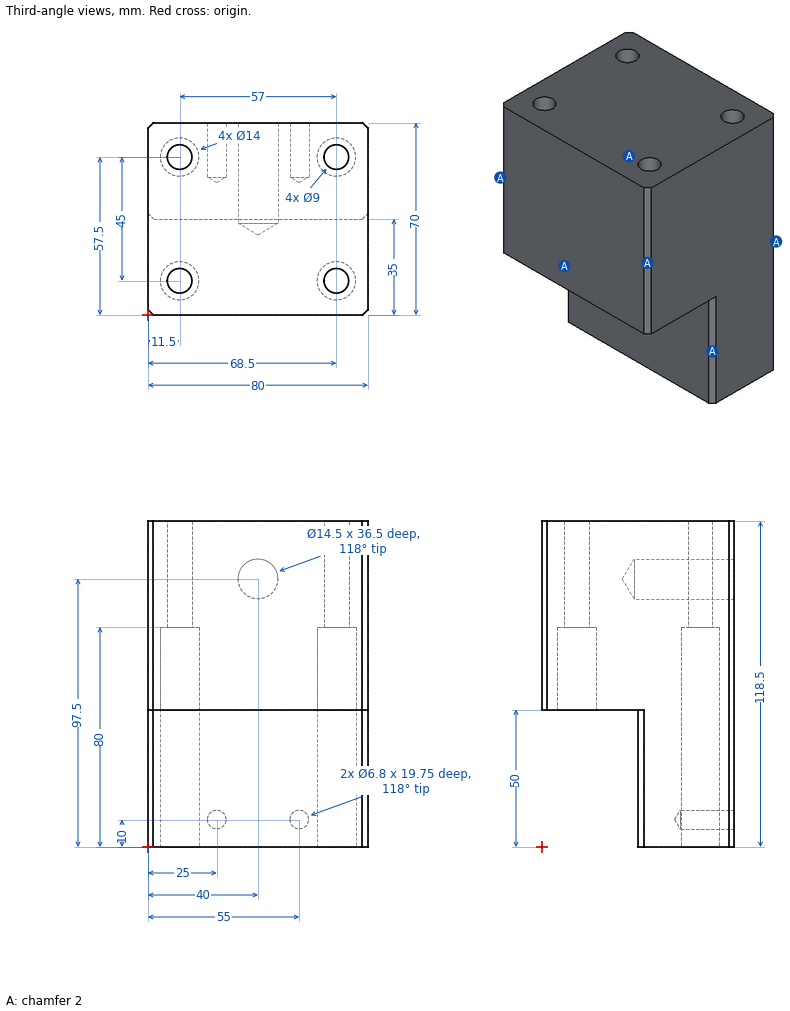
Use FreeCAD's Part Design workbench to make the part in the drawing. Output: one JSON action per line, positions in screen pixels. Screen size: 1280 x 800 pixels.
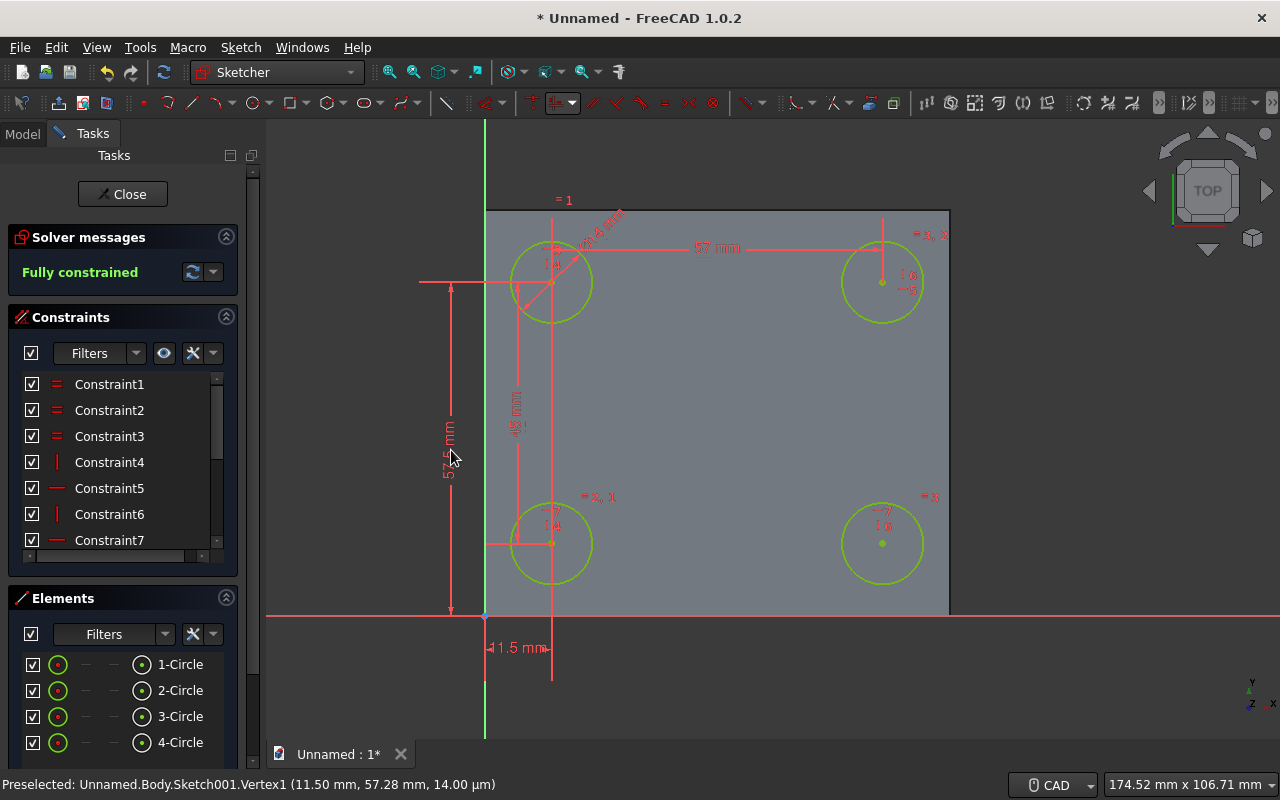
{"action": "left_click", "coordinate": [123, 194]}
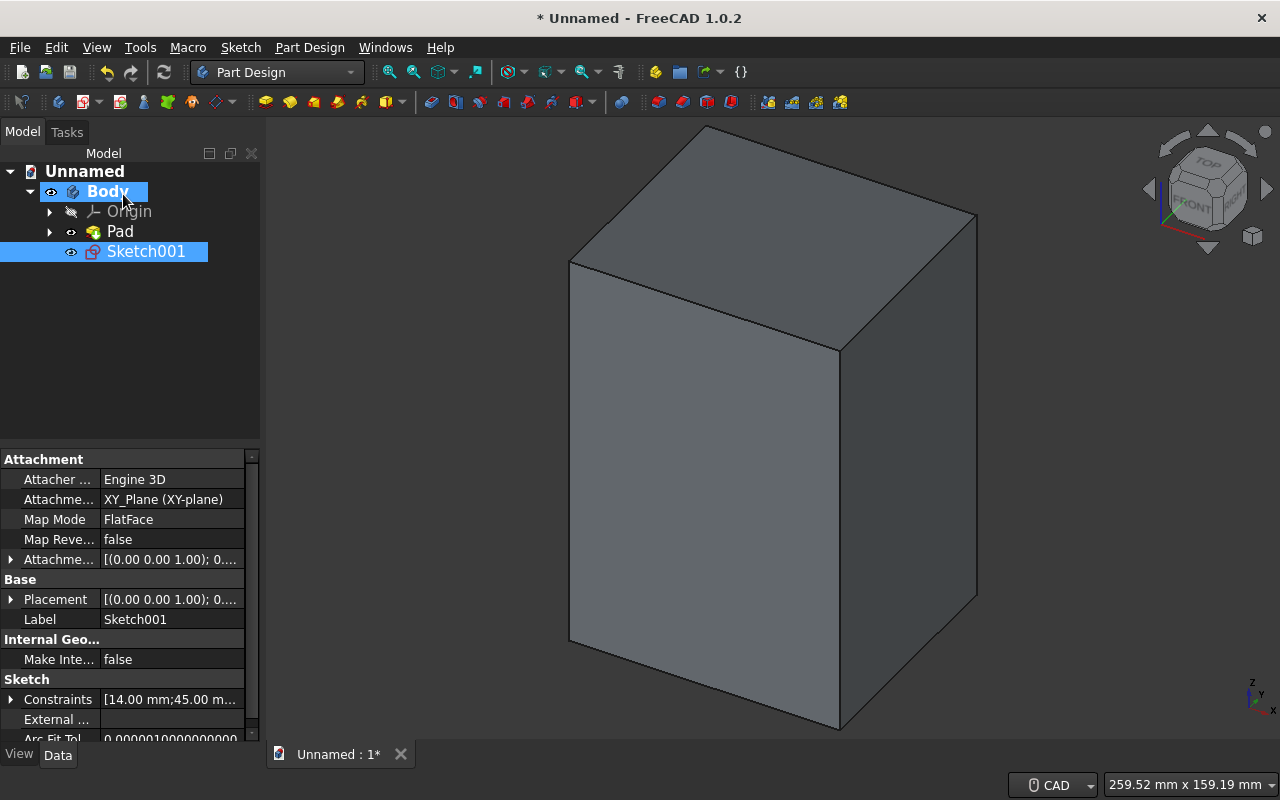
{"action": "left_click", "coordinate": [432, 102]}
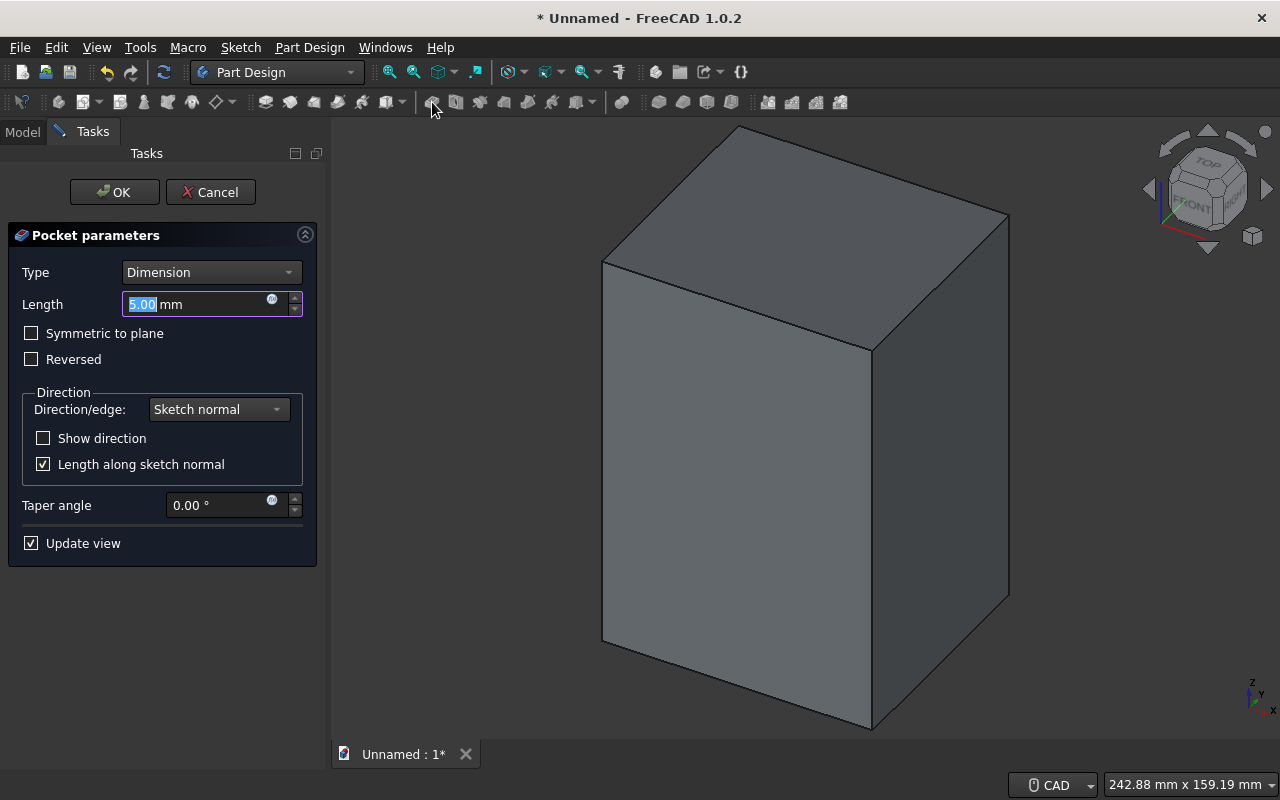
{"action": "type", "text": "80"}
{"action": "key", "text": "Tab"}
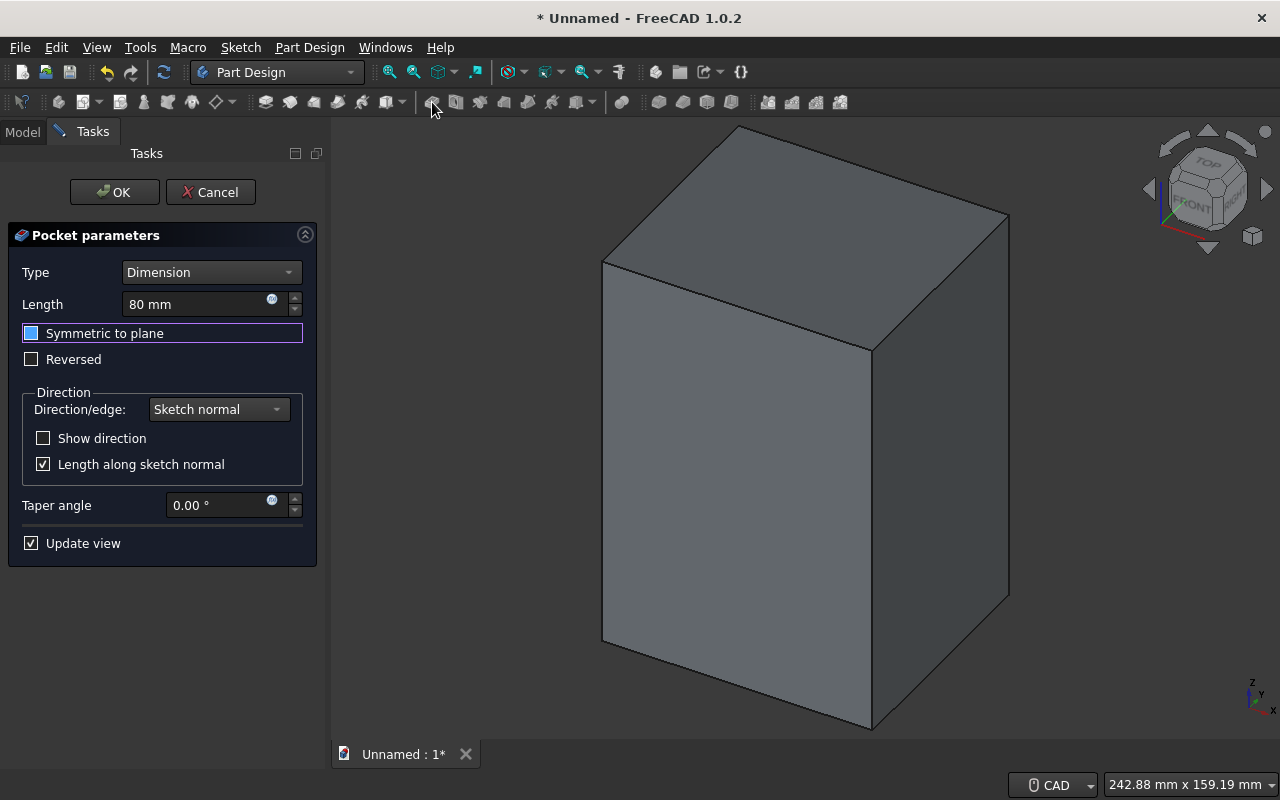
{"action": "left_click", "coordinate": [30, 359]}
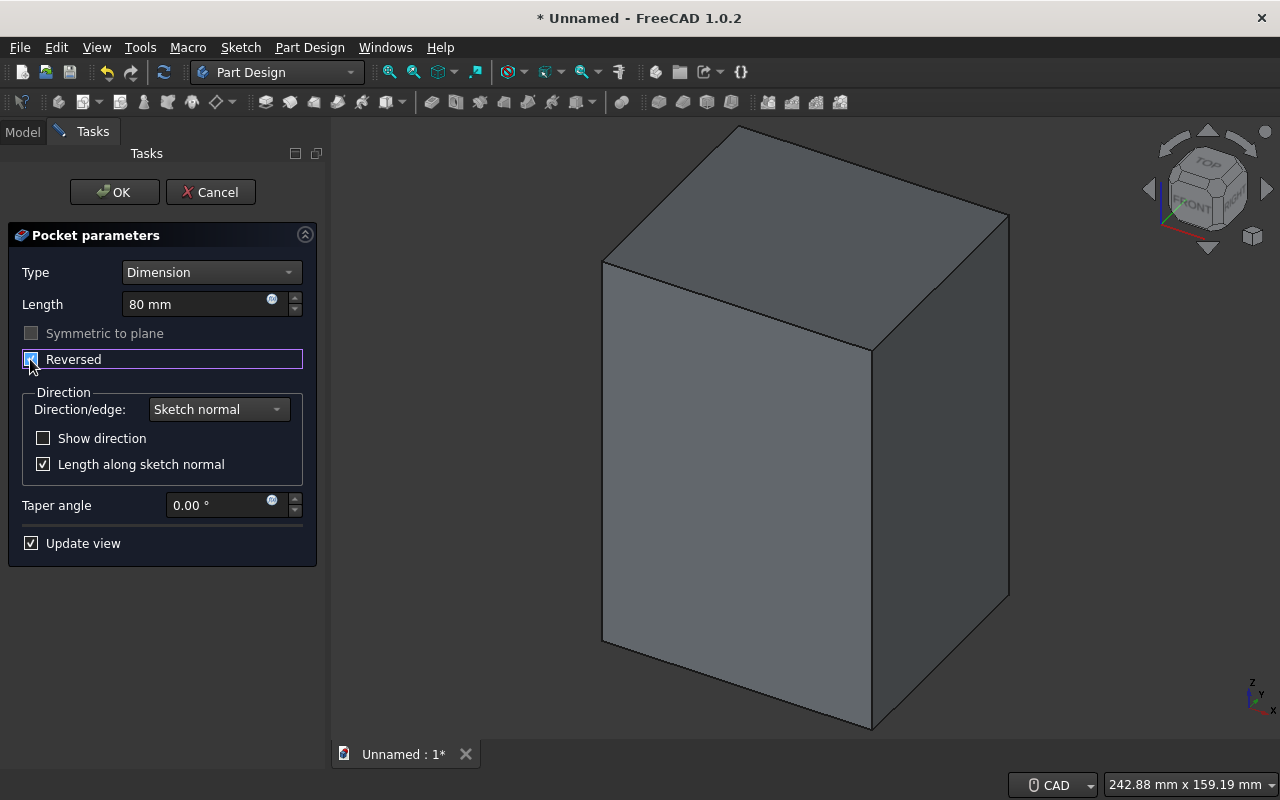
{"action": "left_click", "coordinate": [115, 192]}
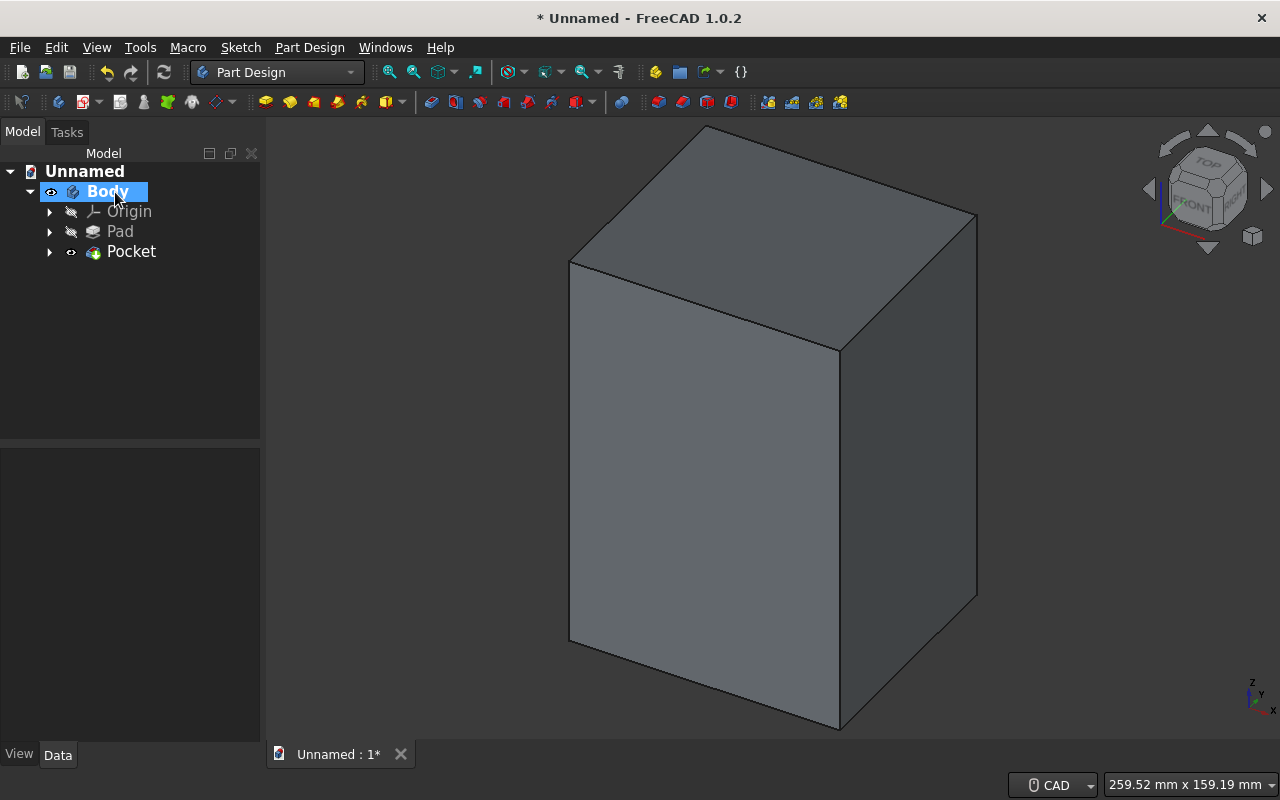
{"action": "left_click", "coordinate": [84, 102]}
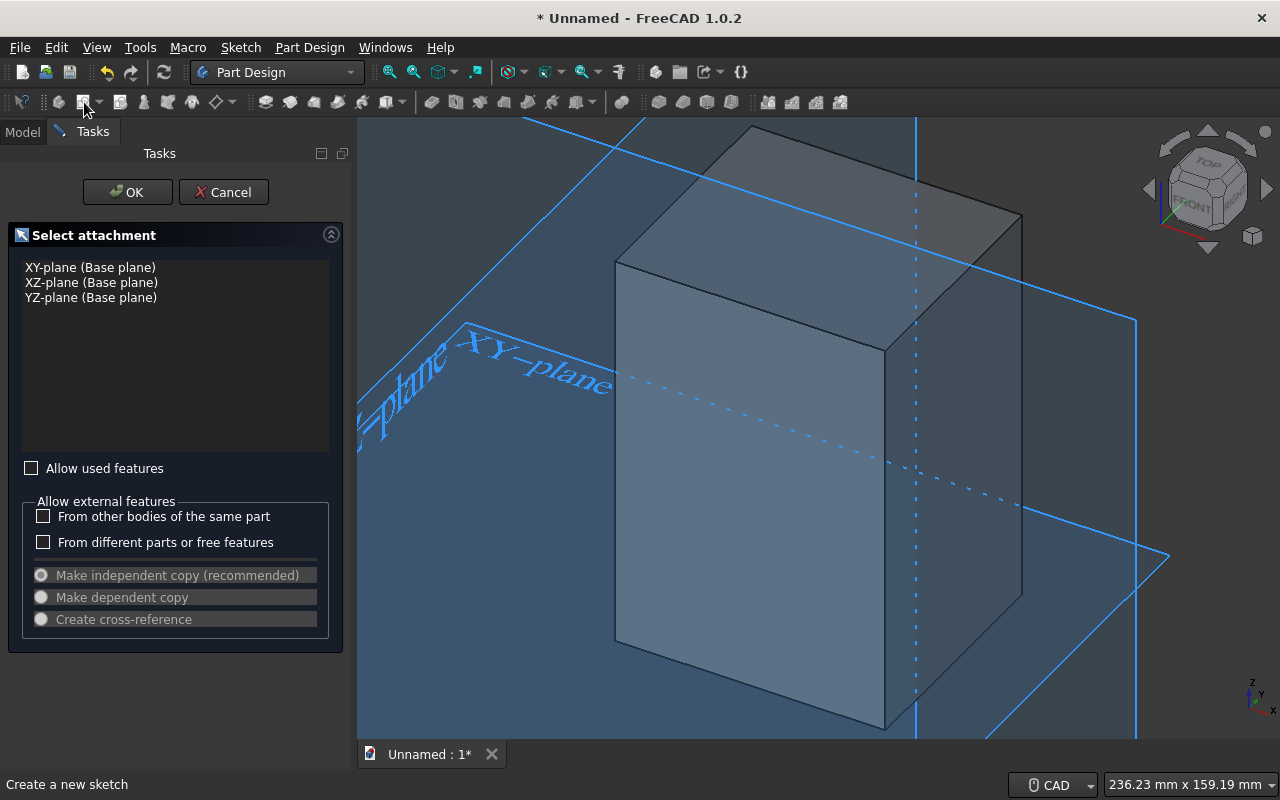
{"action": "left_click", "coordinate": [82, 268]}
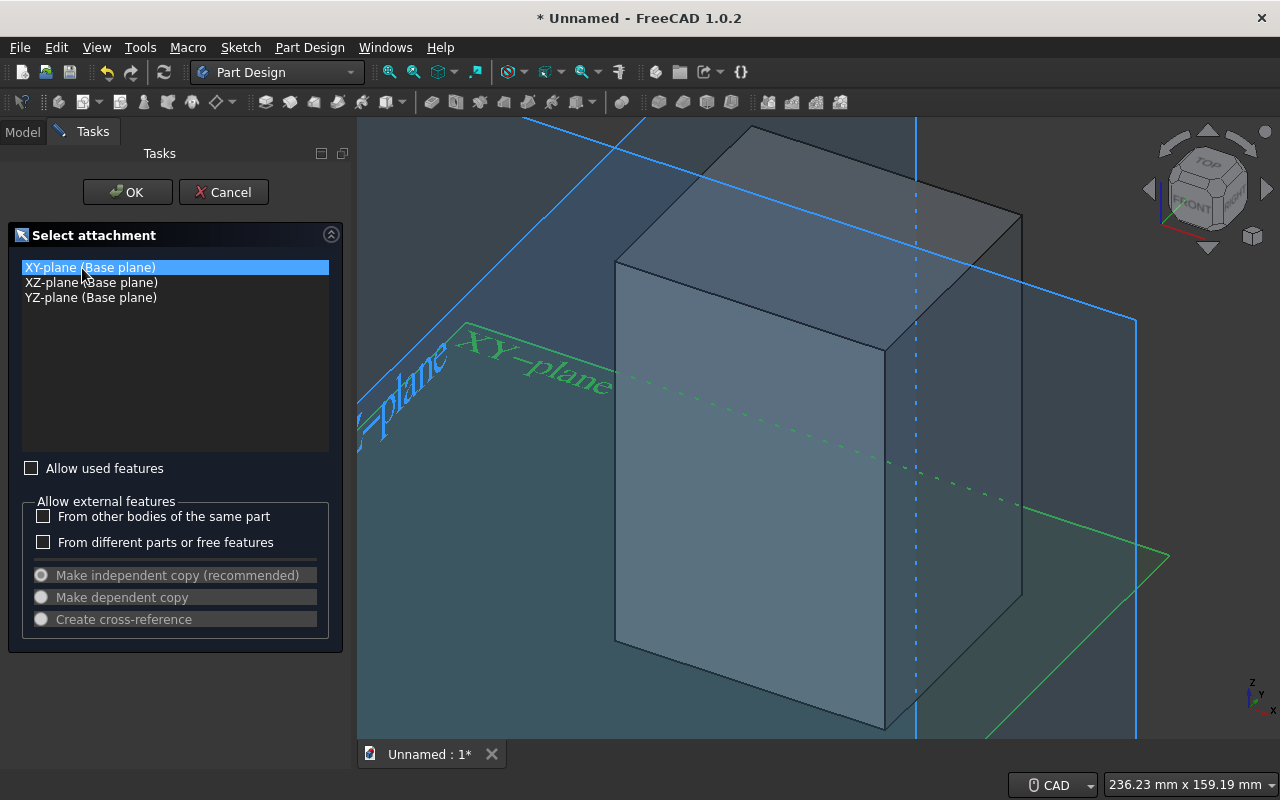
{"action": "left_click", "coordinate": [128, 192]}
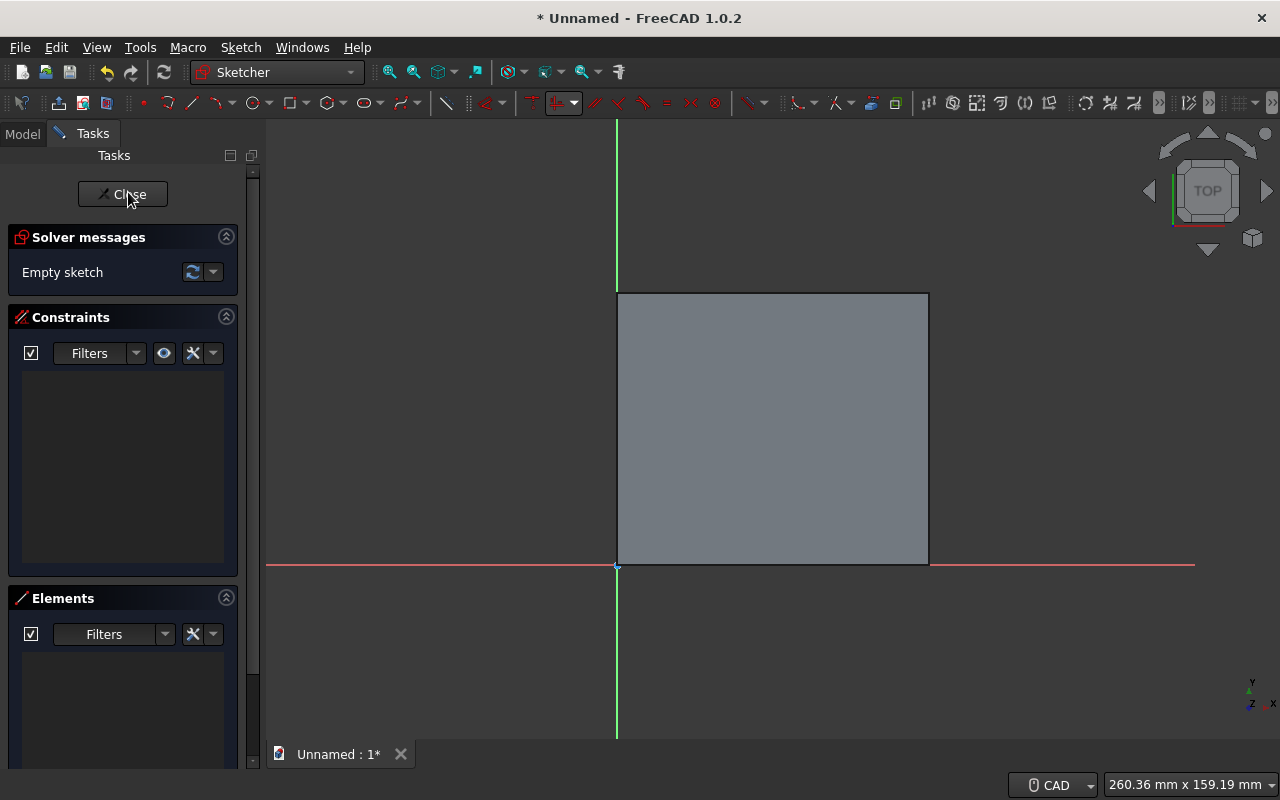
{"action": "key", "text": "q s"}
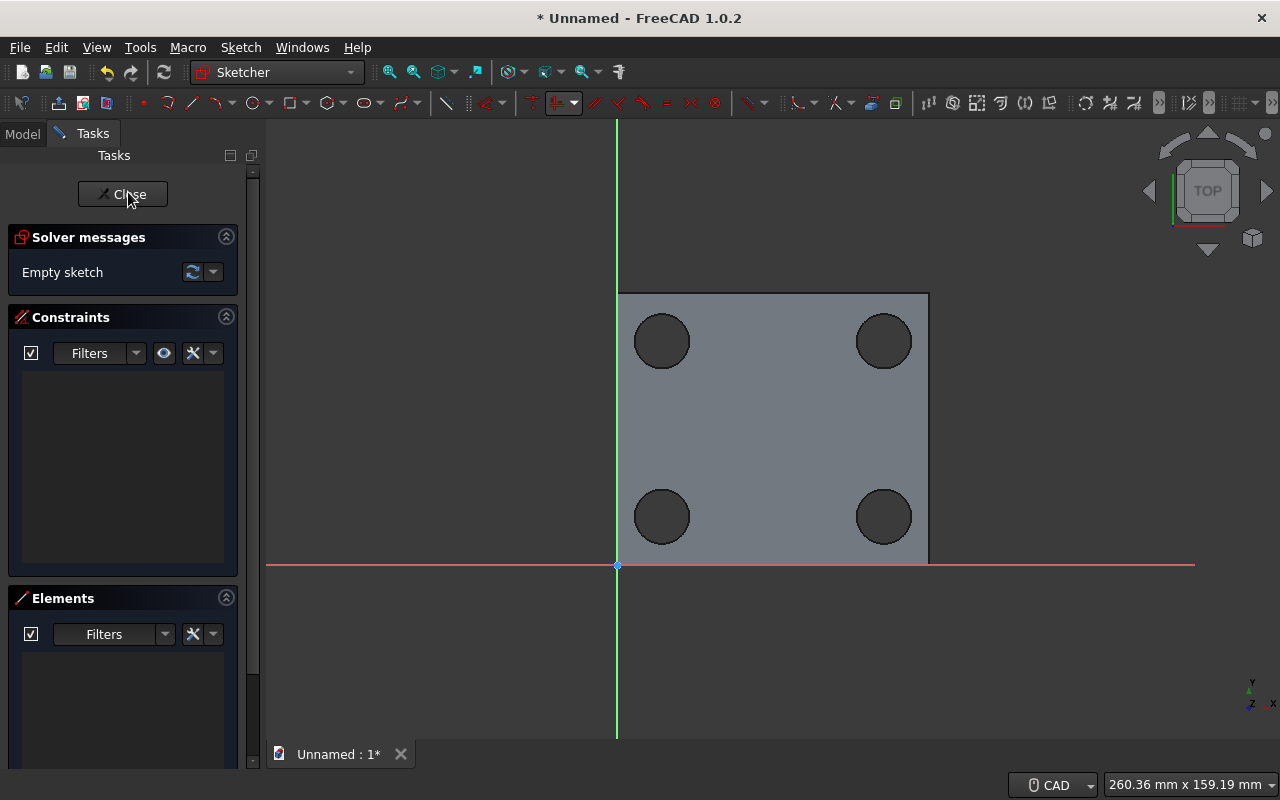
{"action": "scroll", "coordinate": [871, 476], "scroll_direction": "up", "scroll_amount": 2}